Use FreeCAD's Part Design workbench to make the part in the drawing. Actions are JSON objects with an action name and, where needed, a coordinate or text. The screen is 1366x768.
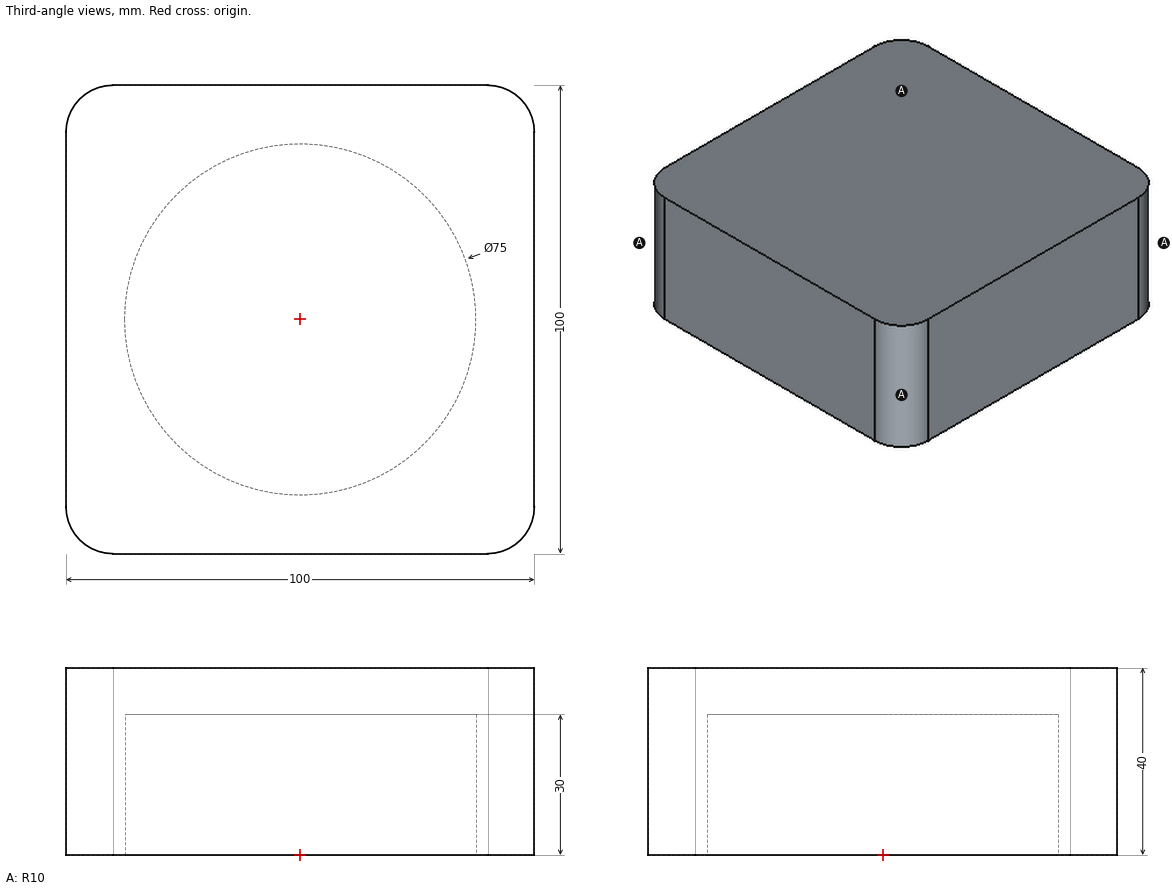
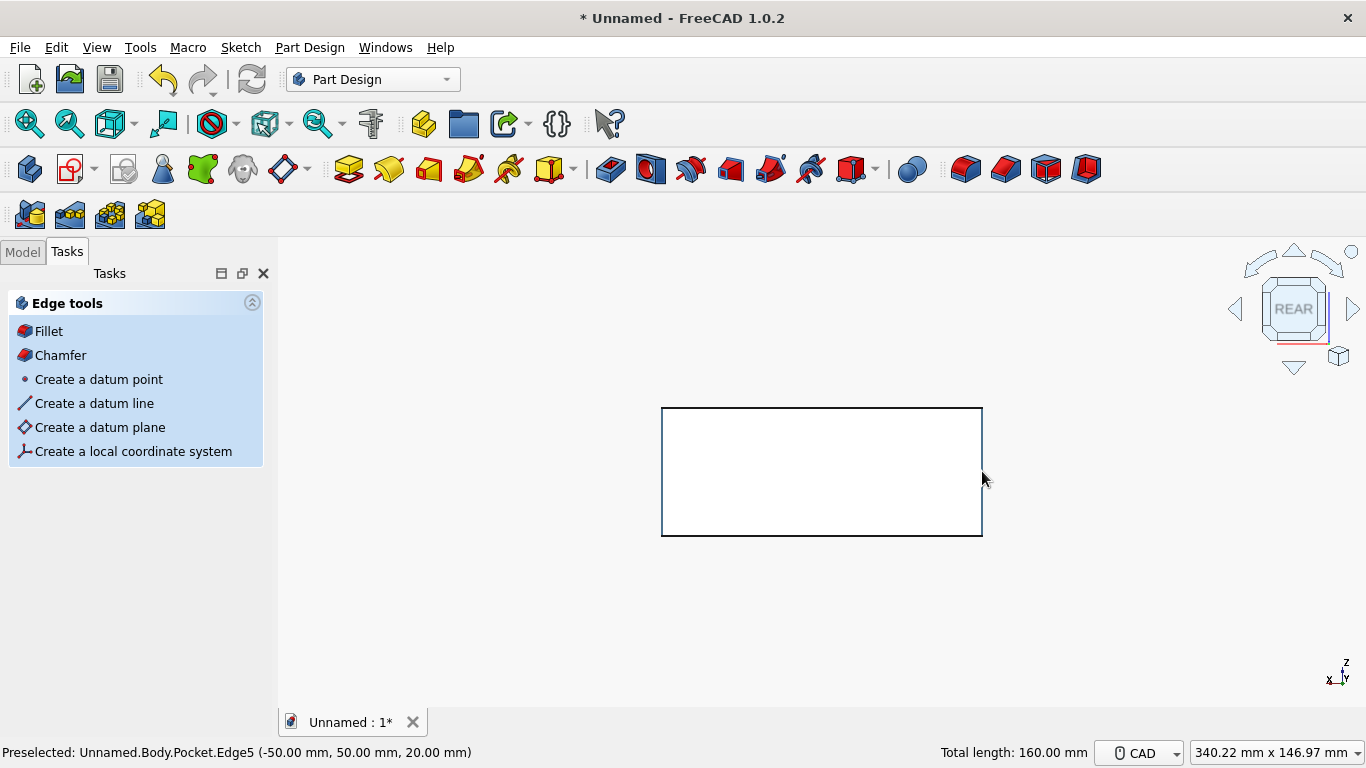
{"action": "left_click", "coordinate": [966, 170]}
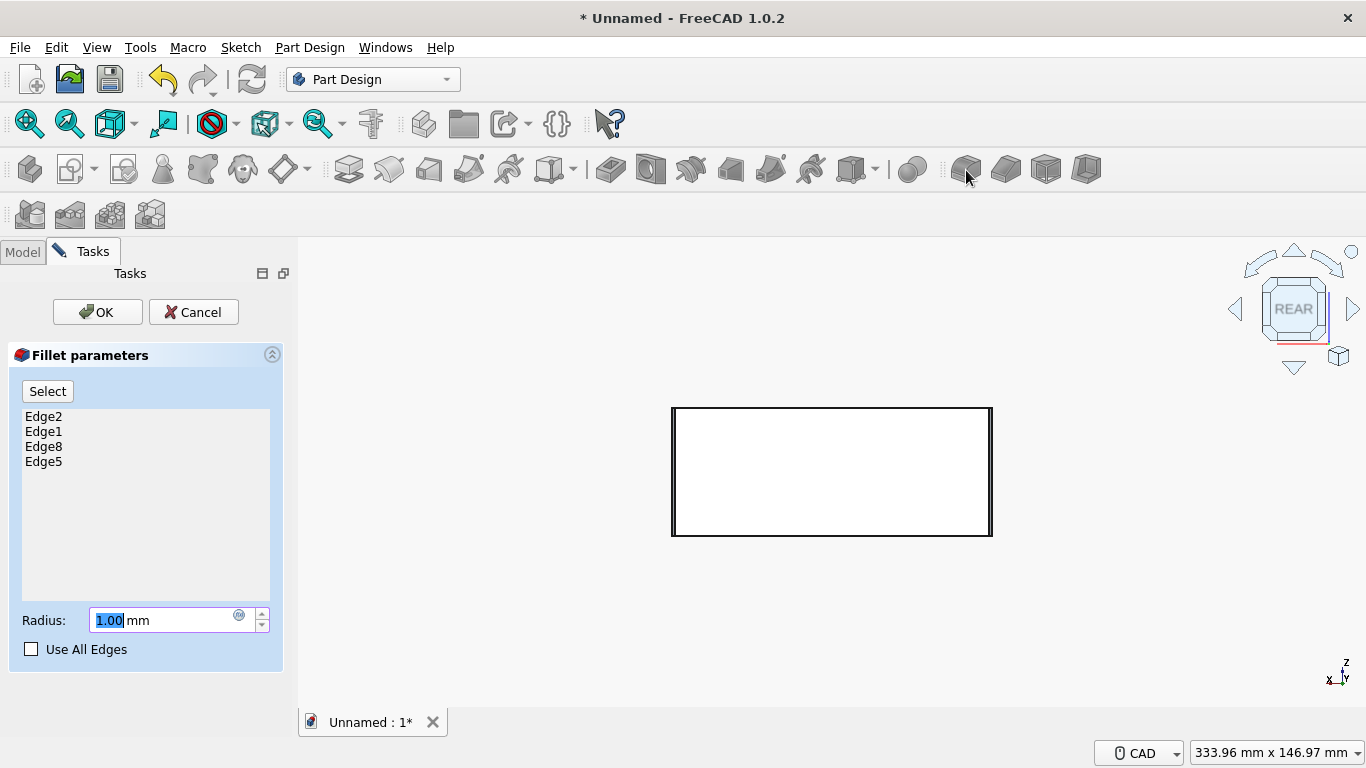
{"action": "type", "text": "10"}
{"action": "key", "text": "Tab"}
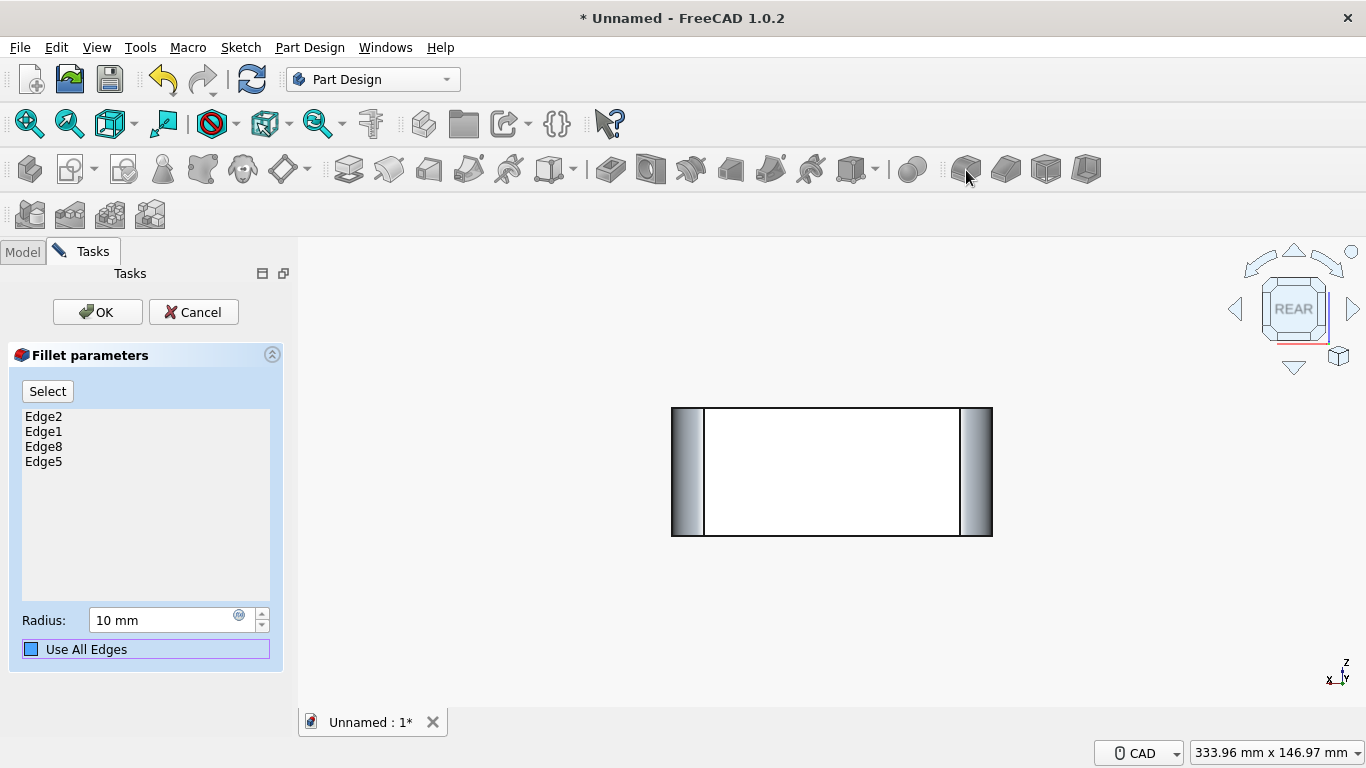
{"action": "left_click", "coordinate": [98, 312]}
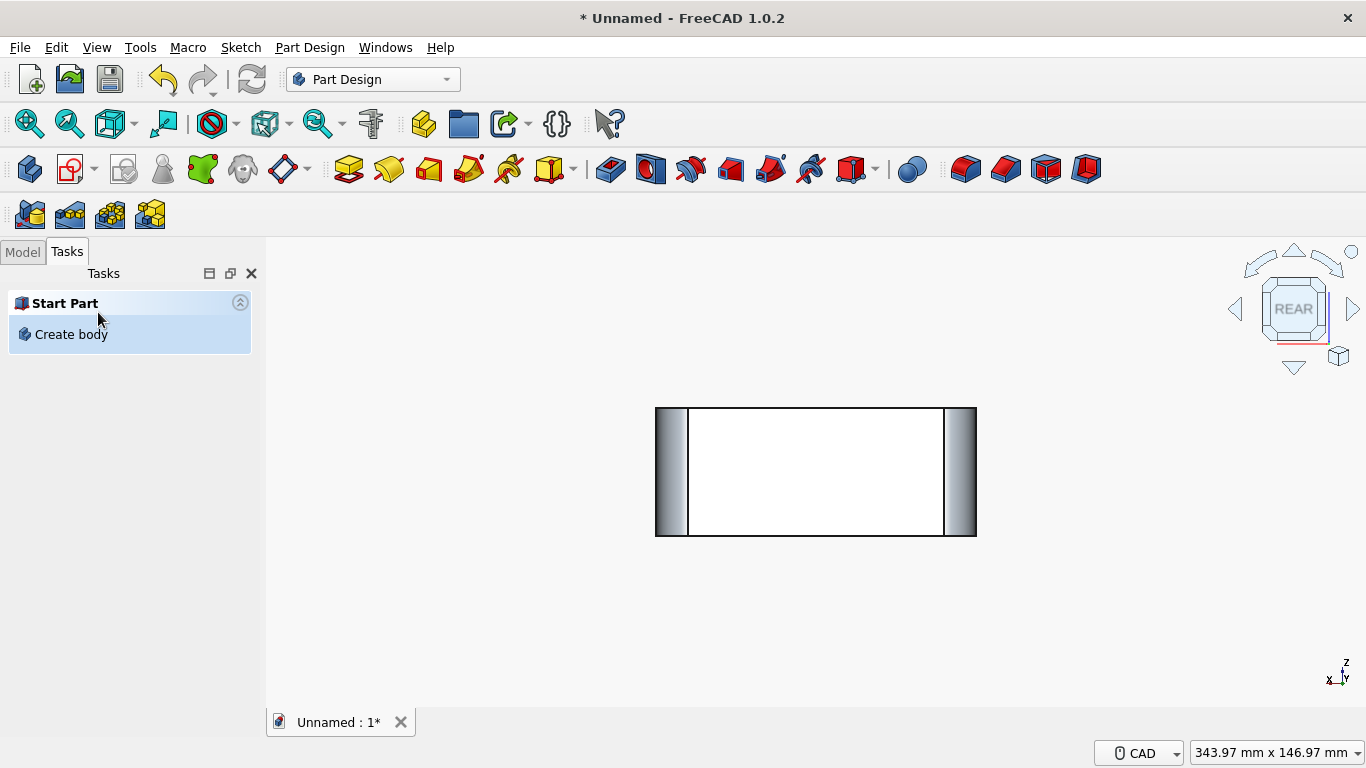
{"action": "key", "text": "0"}